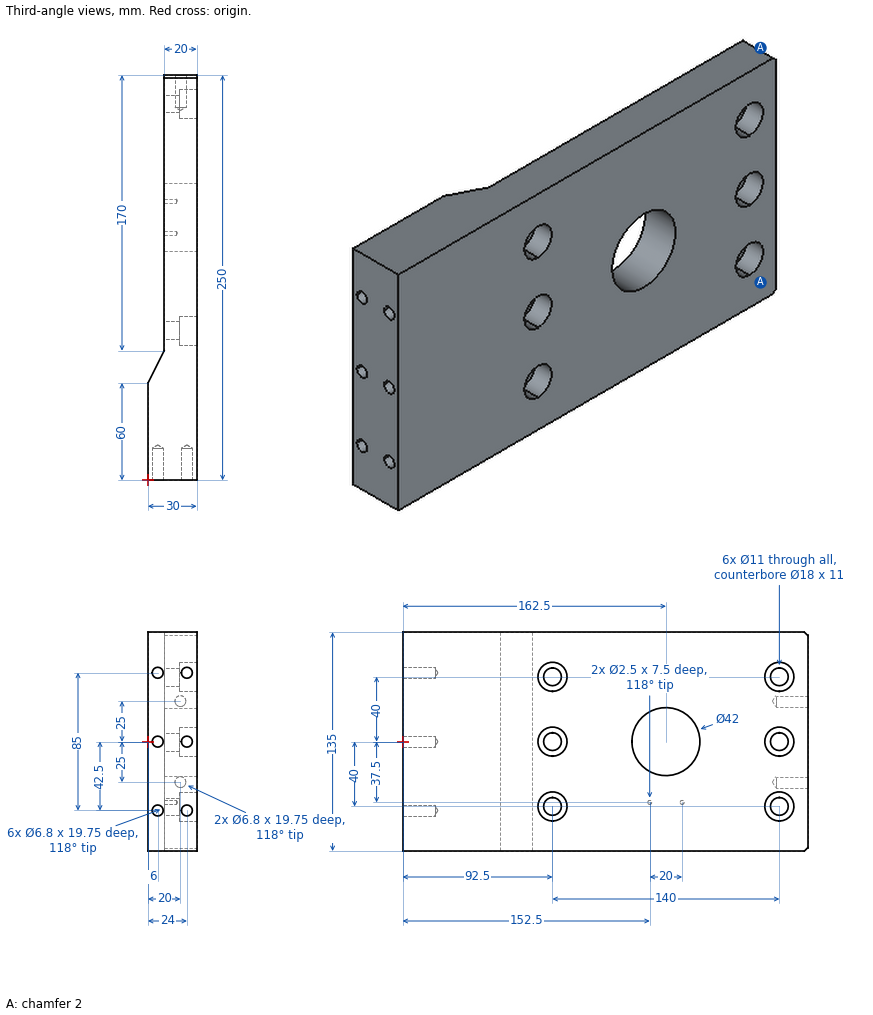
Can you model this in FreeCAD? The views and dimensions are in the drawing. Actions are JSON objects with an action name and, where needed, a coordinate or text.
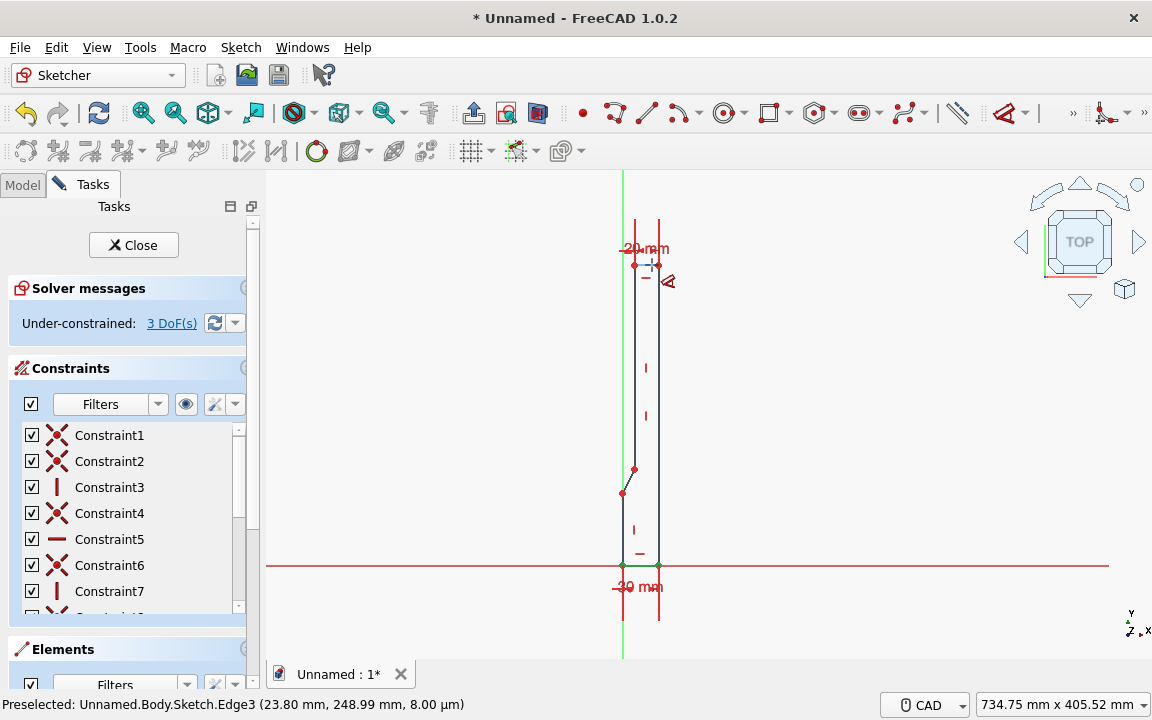
{"action": "left_click", "coordinate": [623, 515]}
{"action": "left_click", "coordinate": [589, 530]}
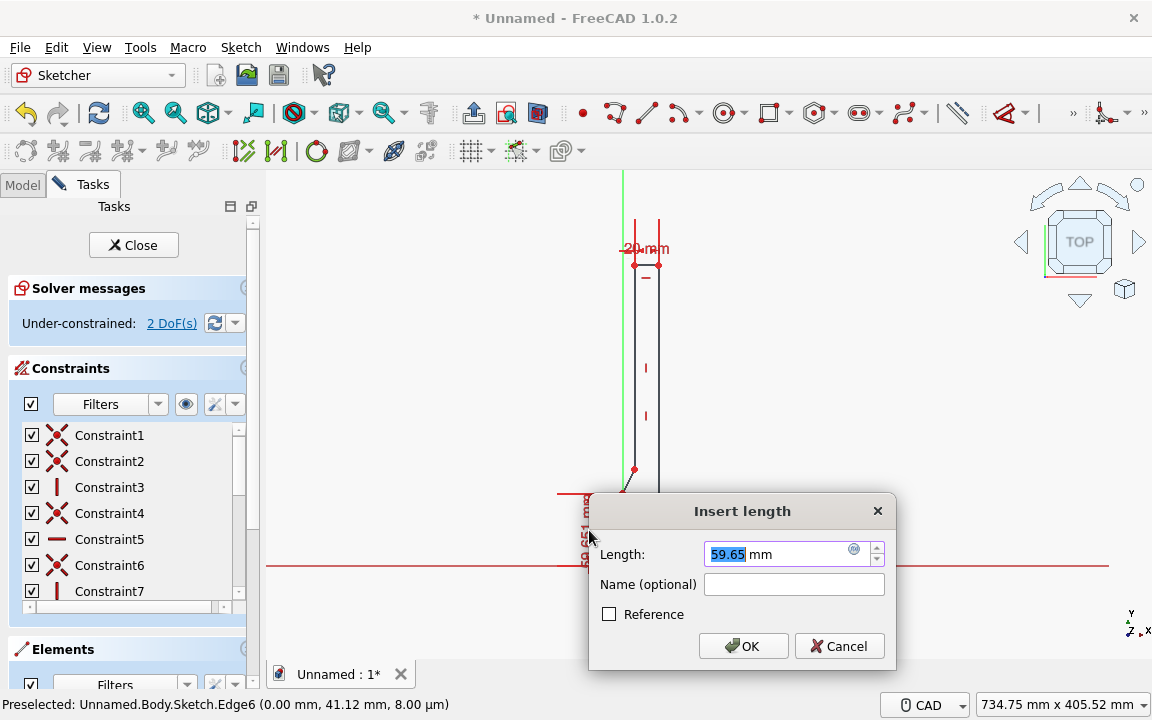
{"action": "type", "text": "60"}
{"action": "key", "text": "Return"}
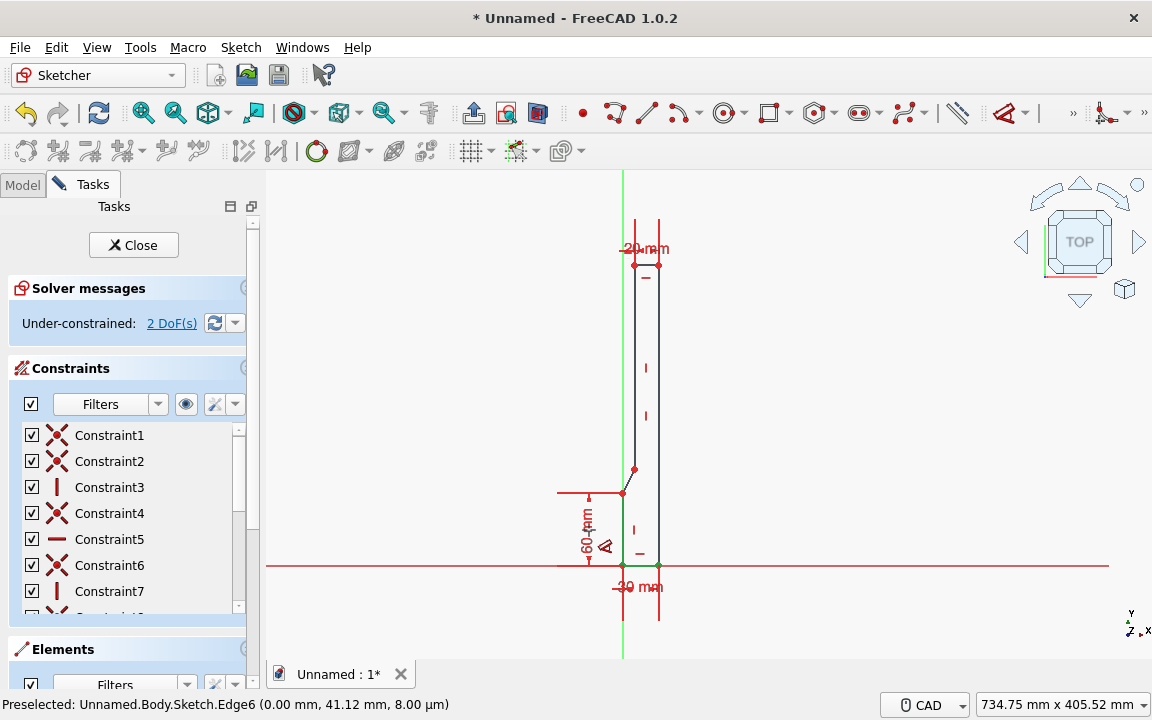
{"action": "left_click", "coordinate": [659, 476]}
{"action": "left_click", "coordinate": [693, 415]}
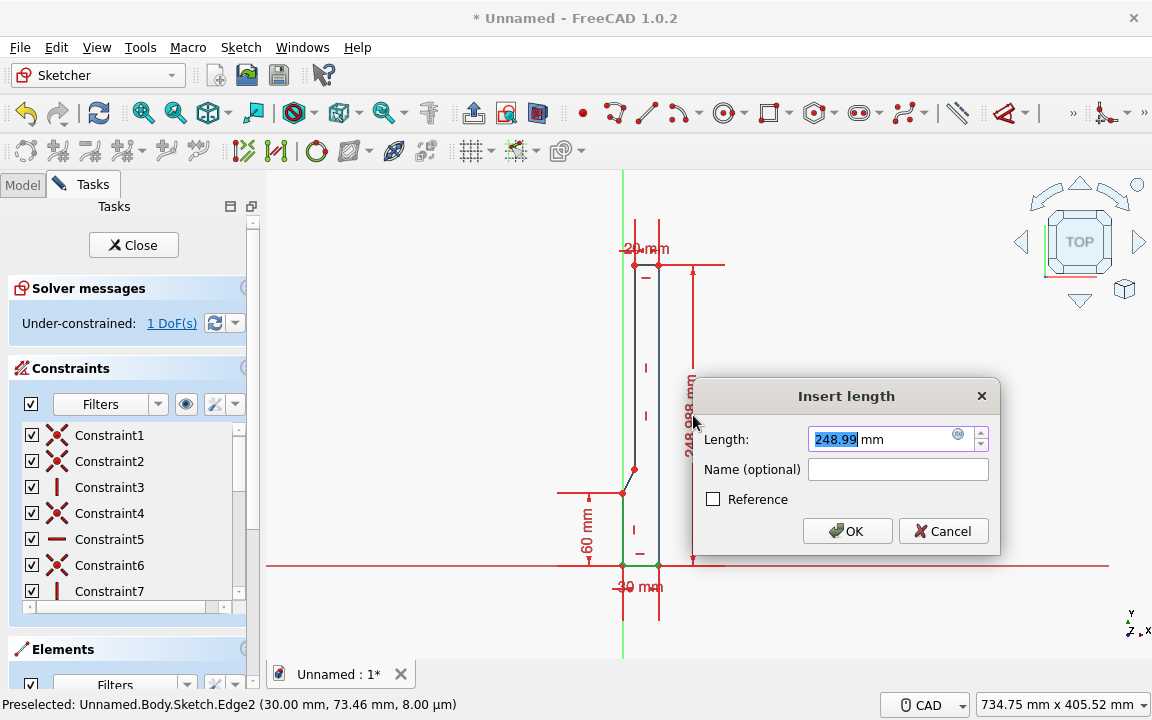
{"action": "type", "text": "250"}
{"action": "key", "text": "Return"}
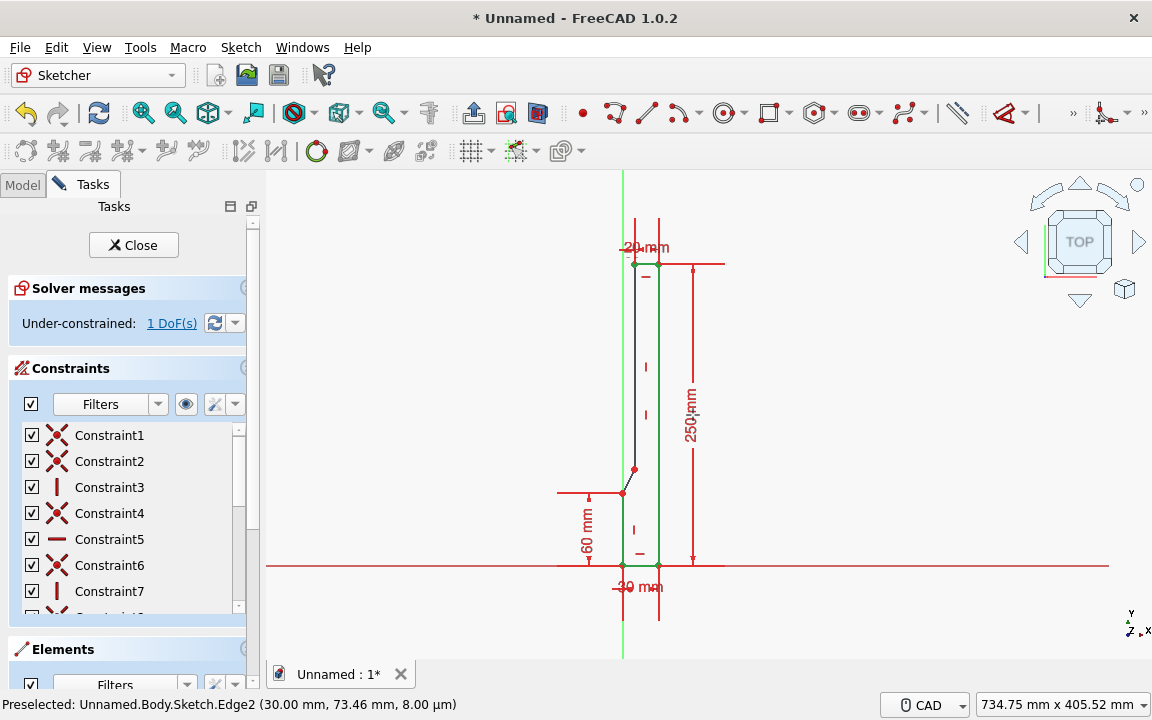
{"action": "left_click", "coordinate": [635, 326]}
{"action": "left_click", "coordinate": [601, 367]}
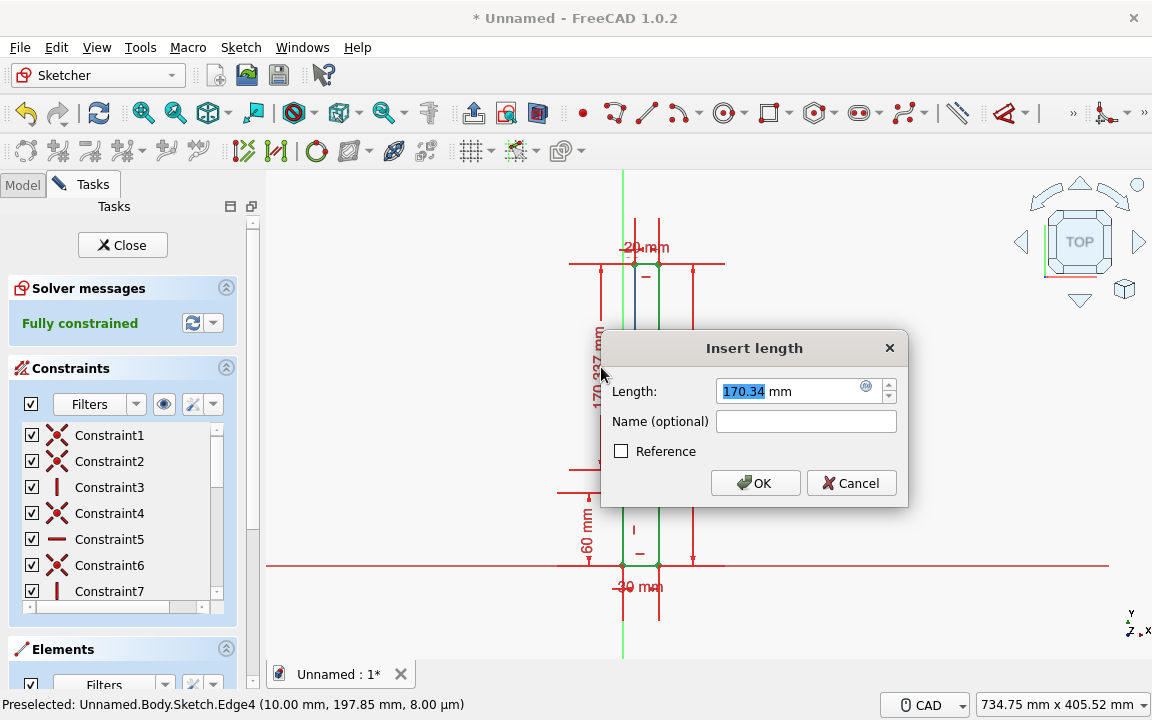
{"action": "type", "text": "170"}
{"action": "key", "text": "Return"}
{"action": "key", "text": "Escape"}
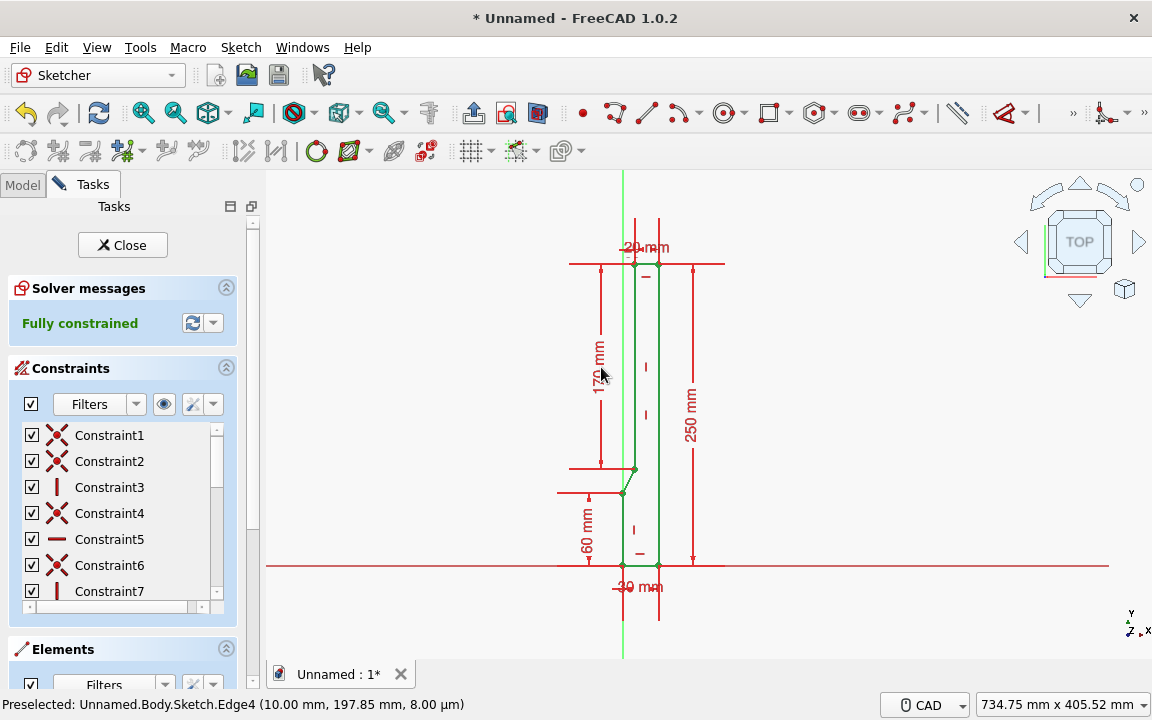
{"action": "left_click", "coordinate": [123, 245]}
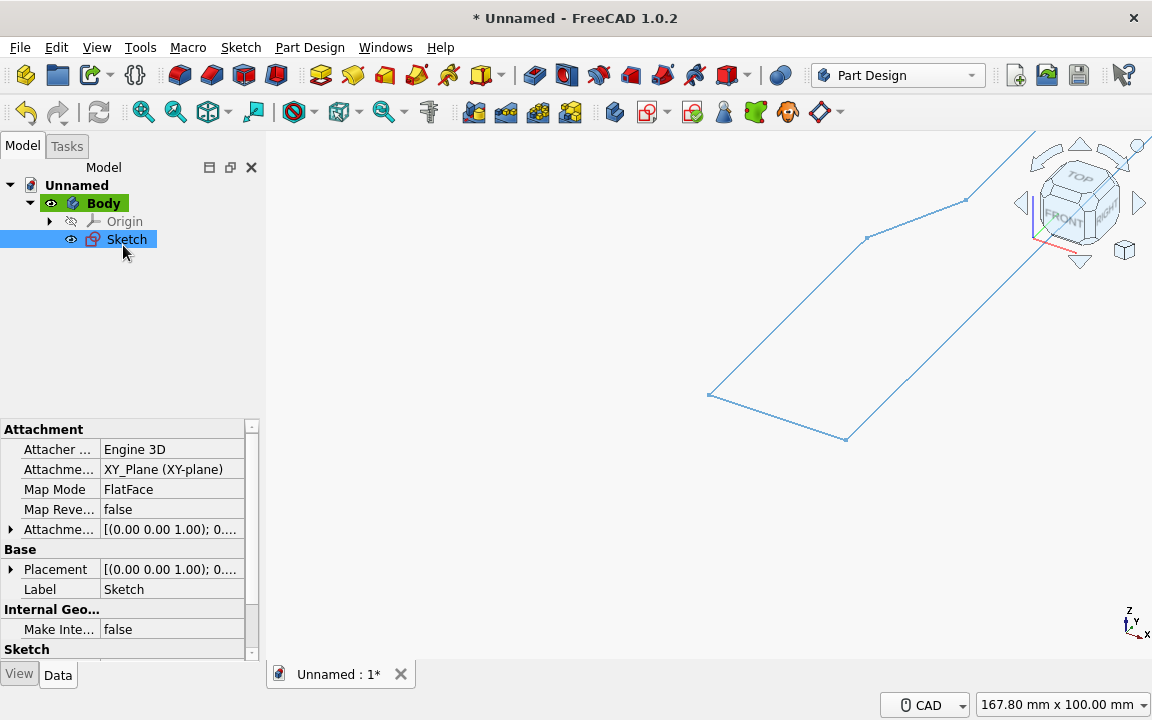
{"action": "left_click", "coordinate": [322, 76]}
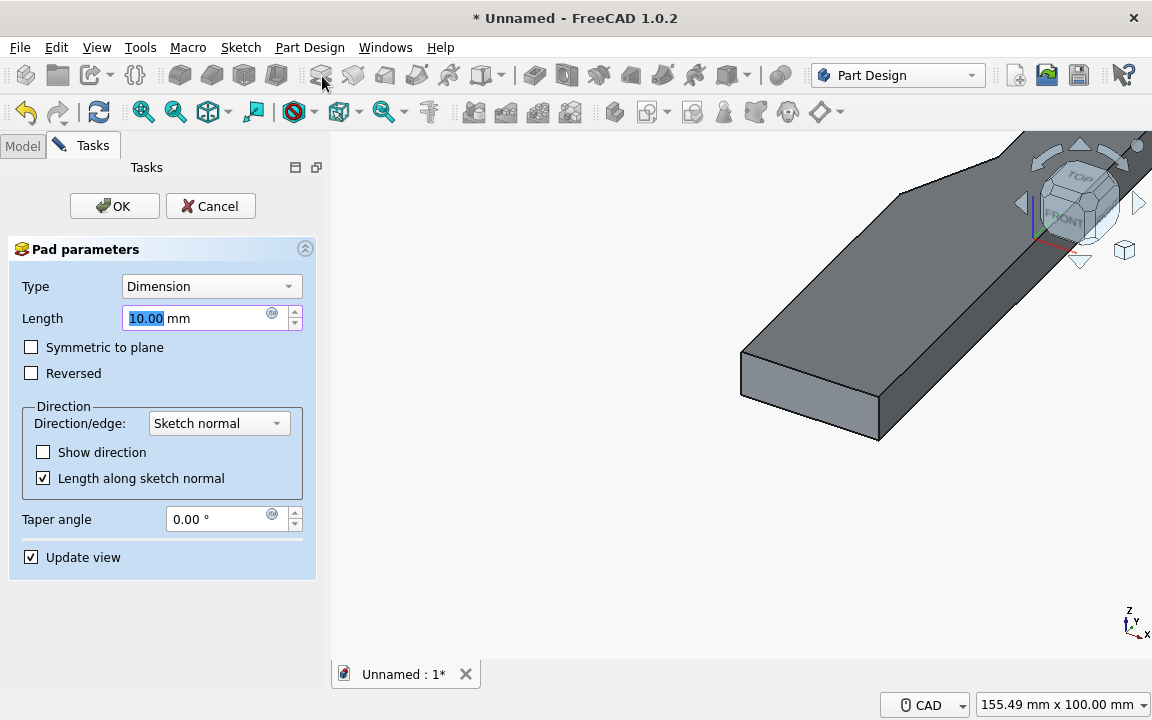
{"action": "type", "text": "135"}
{"action": "key", "text": "Tab"}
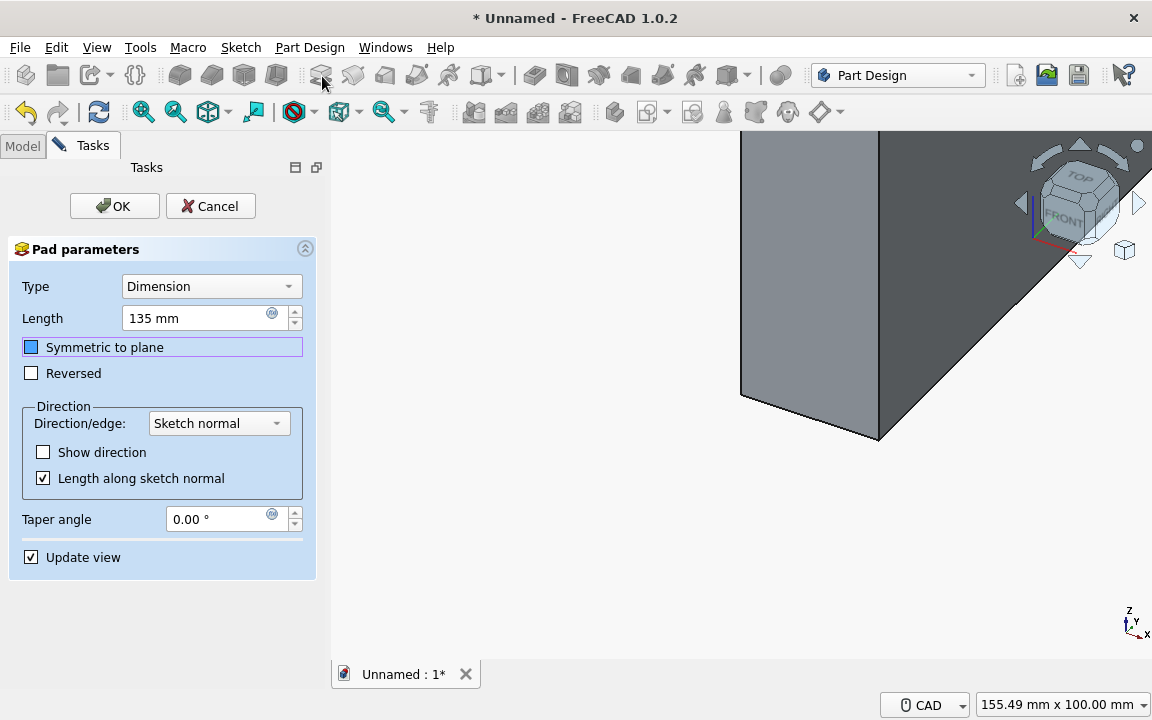
{"action": "left_click", "coordinate": [30, 347]}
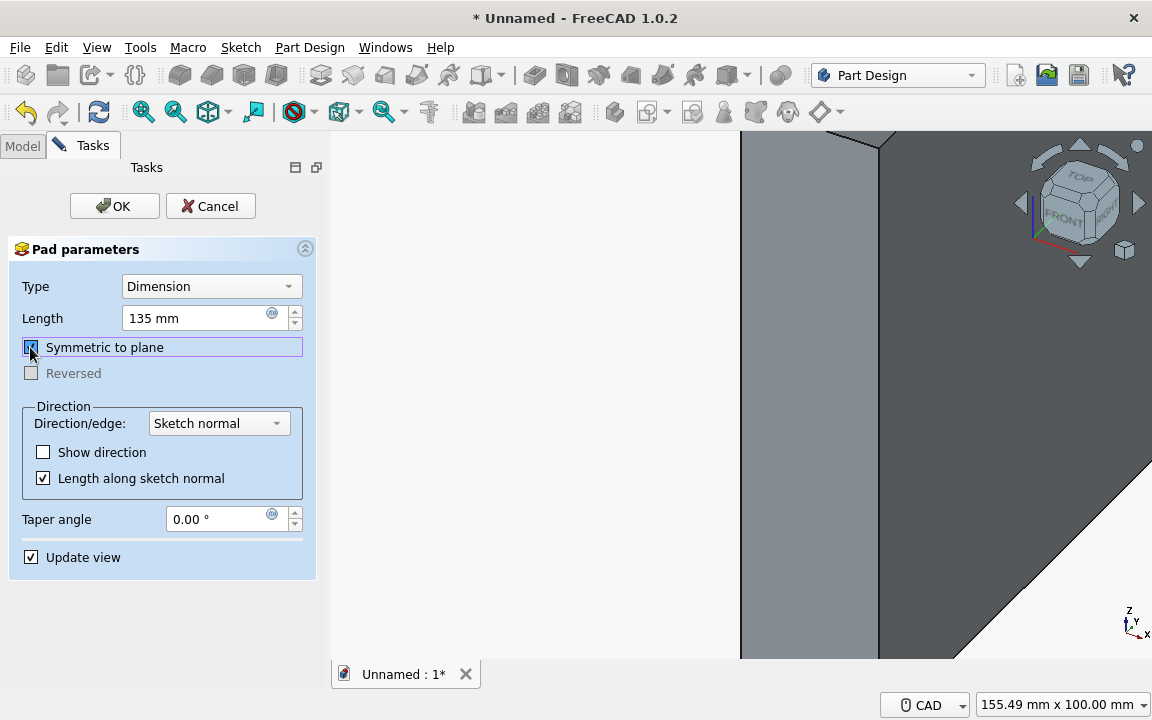
{"action": "left_click", "coordinate": [115, 206]}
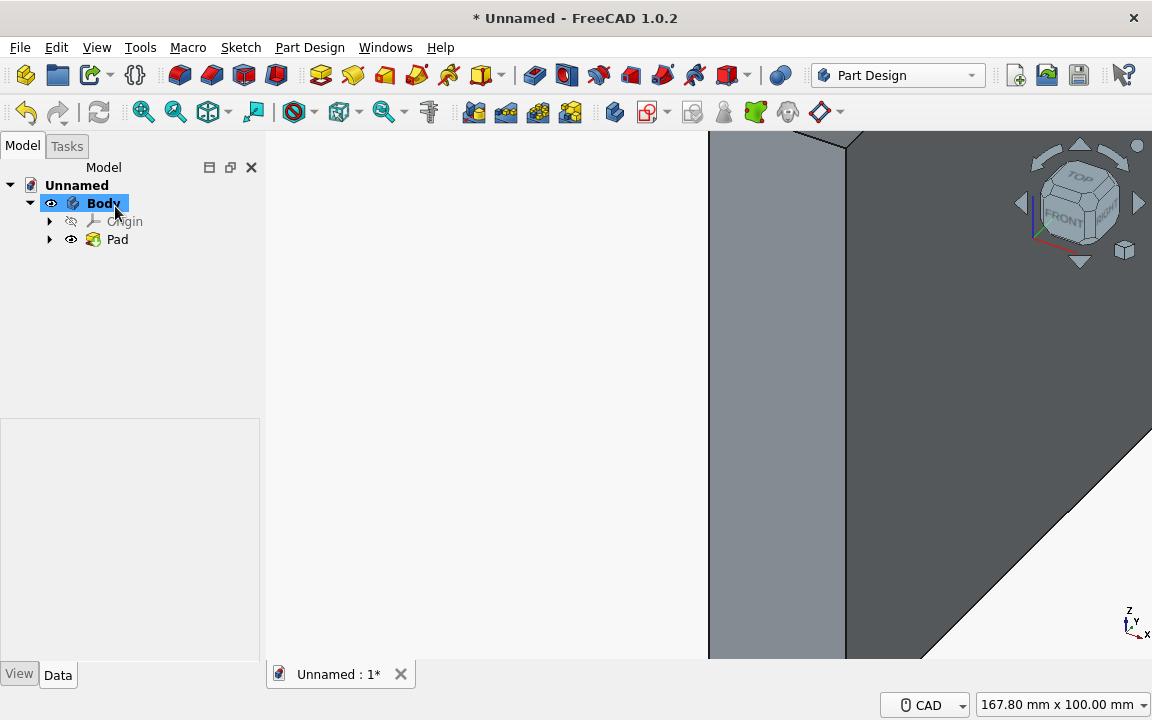
{"action": "left_click", "coordinate": [144, 112]}